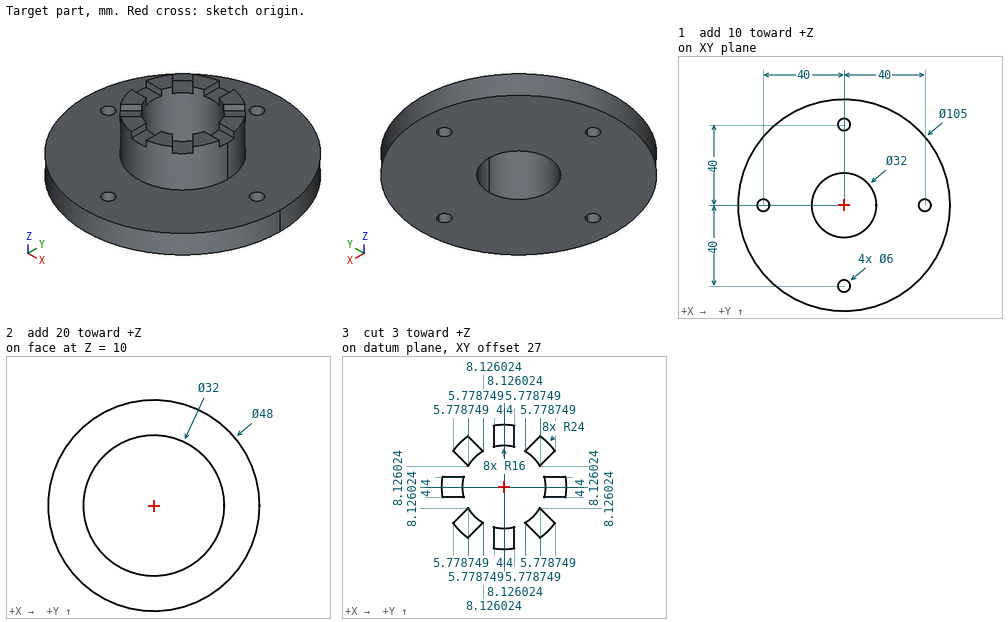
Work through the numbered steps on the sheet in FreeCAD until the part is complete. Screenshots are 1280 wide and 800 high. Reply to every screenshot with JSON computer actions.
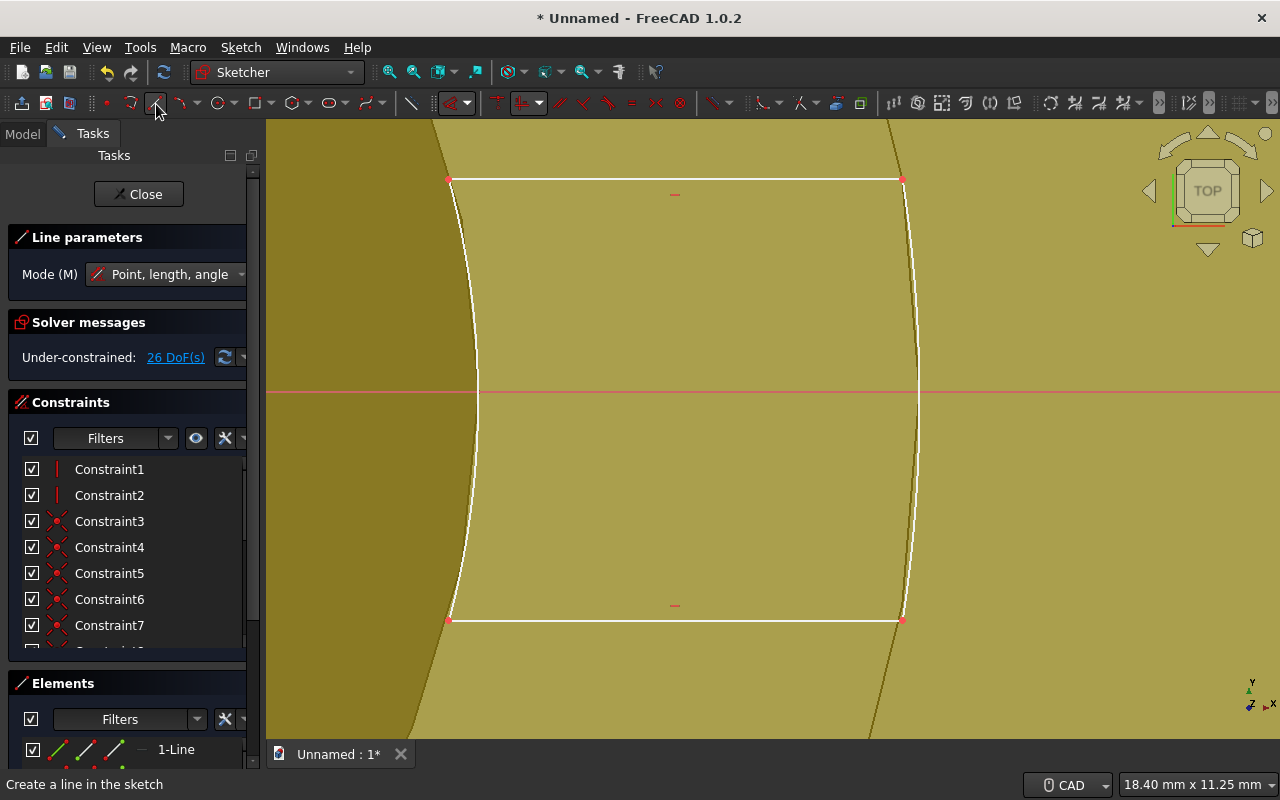
{"action": "scroll", "coordinate": [924, 436], "scroll_direction": "down", "scroll_amount": 9}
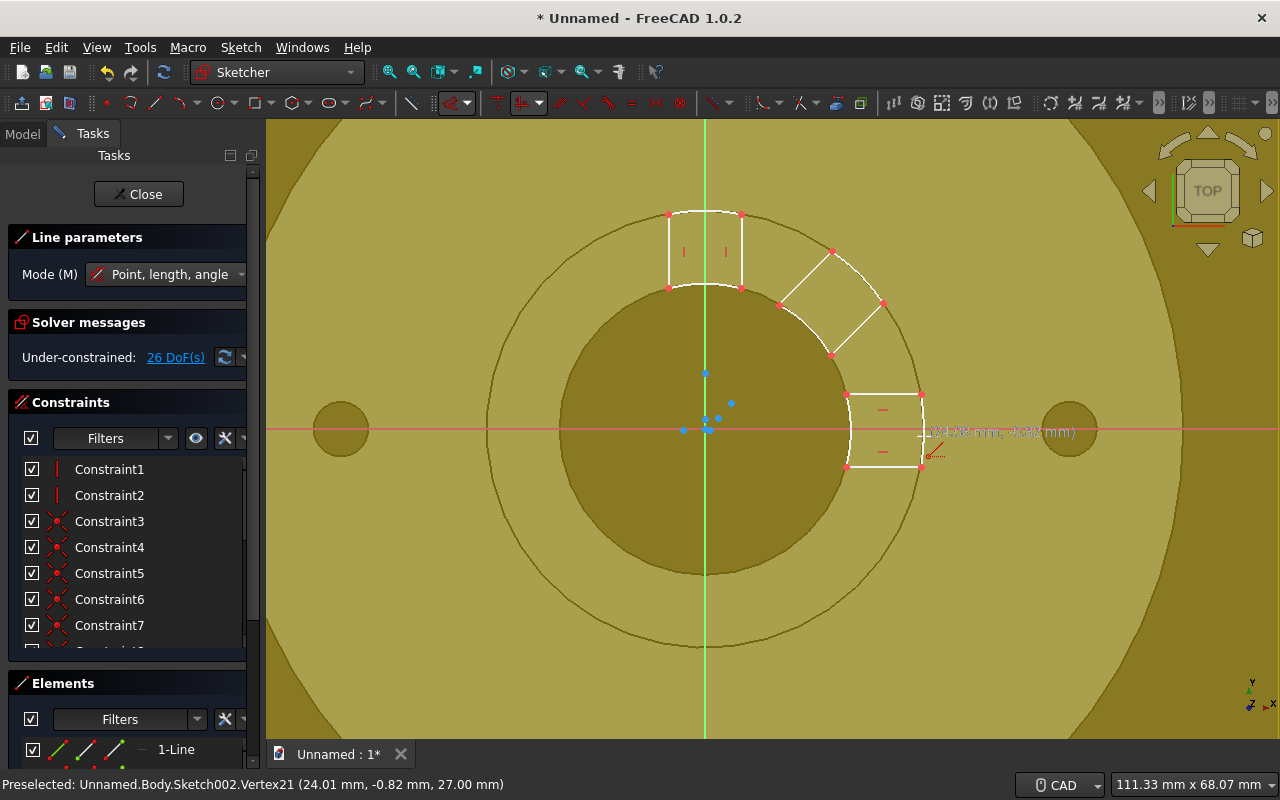
{"action": "left_click", "coordinate": [883, 556]}
{"action": "left_click", "coordinate": [831, 503]}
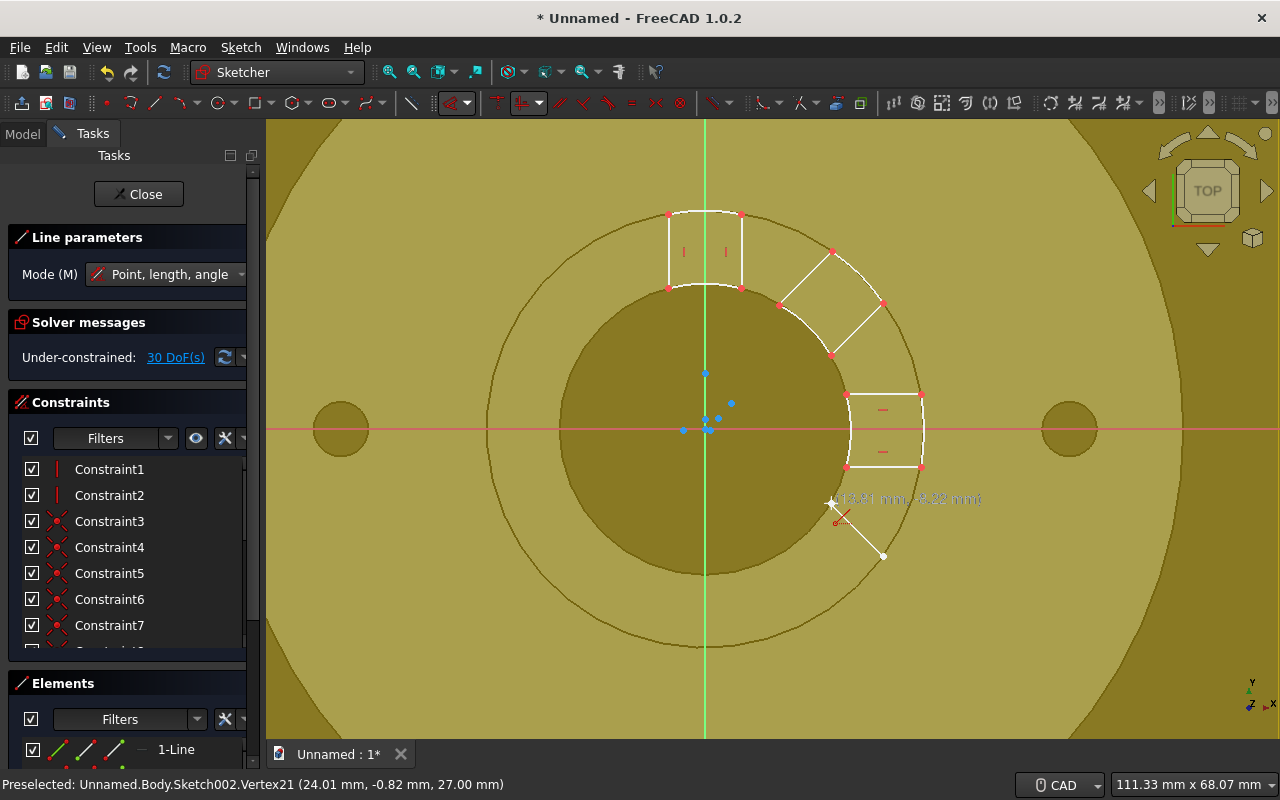
{"action": "left_click", "coordinate": [779, 555]}
{"action": "left_click", "coordinate": [832, 607]}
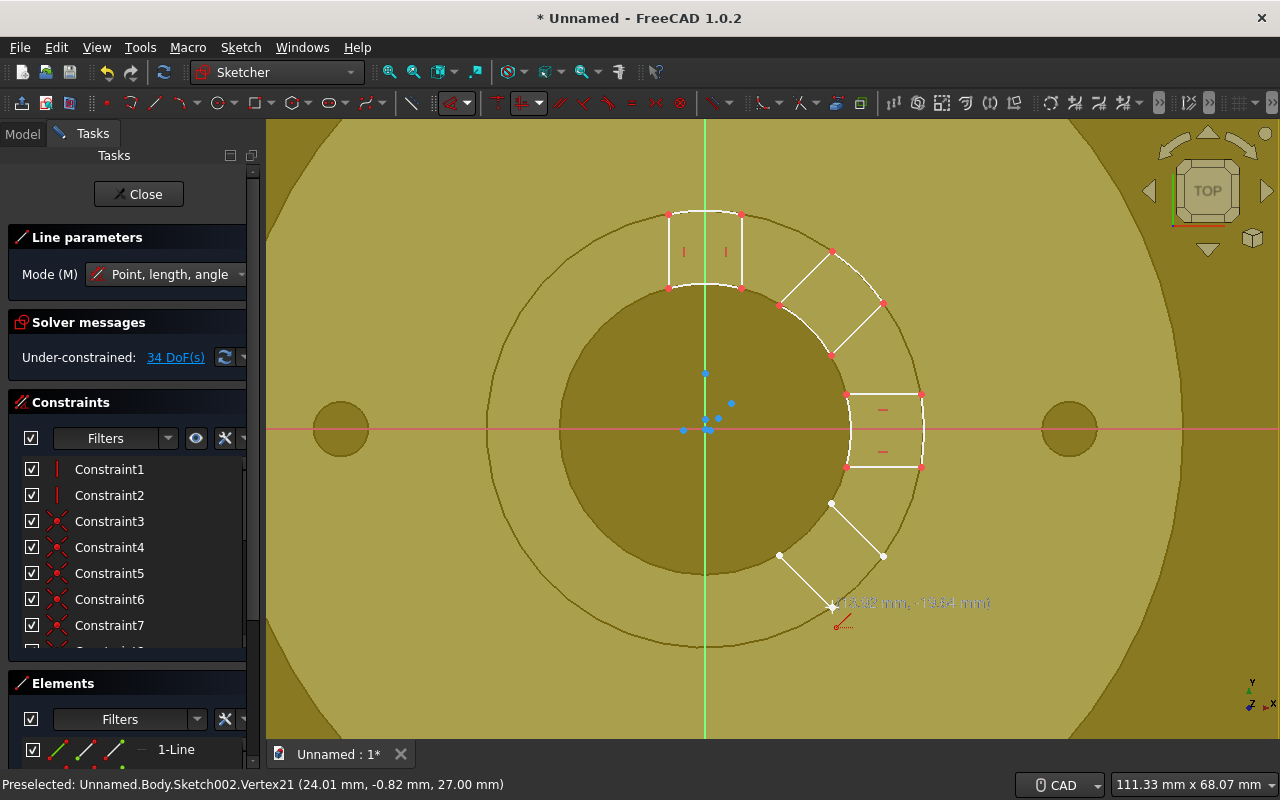
{"action": "left_click", "coordinate": [180, 104]}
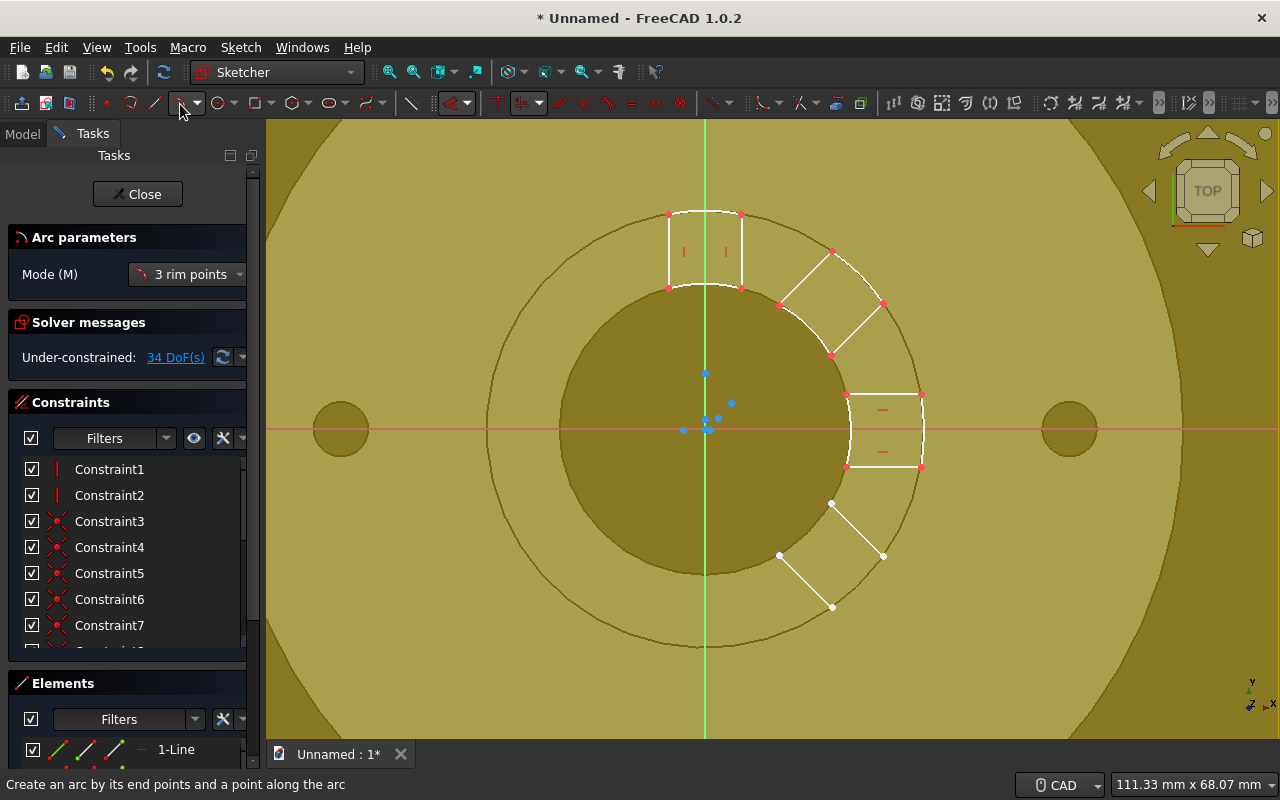
{"action": "left_click", "coordinate": [831, 504]}
{"action": "left_click", "coordinate": [779, 556]}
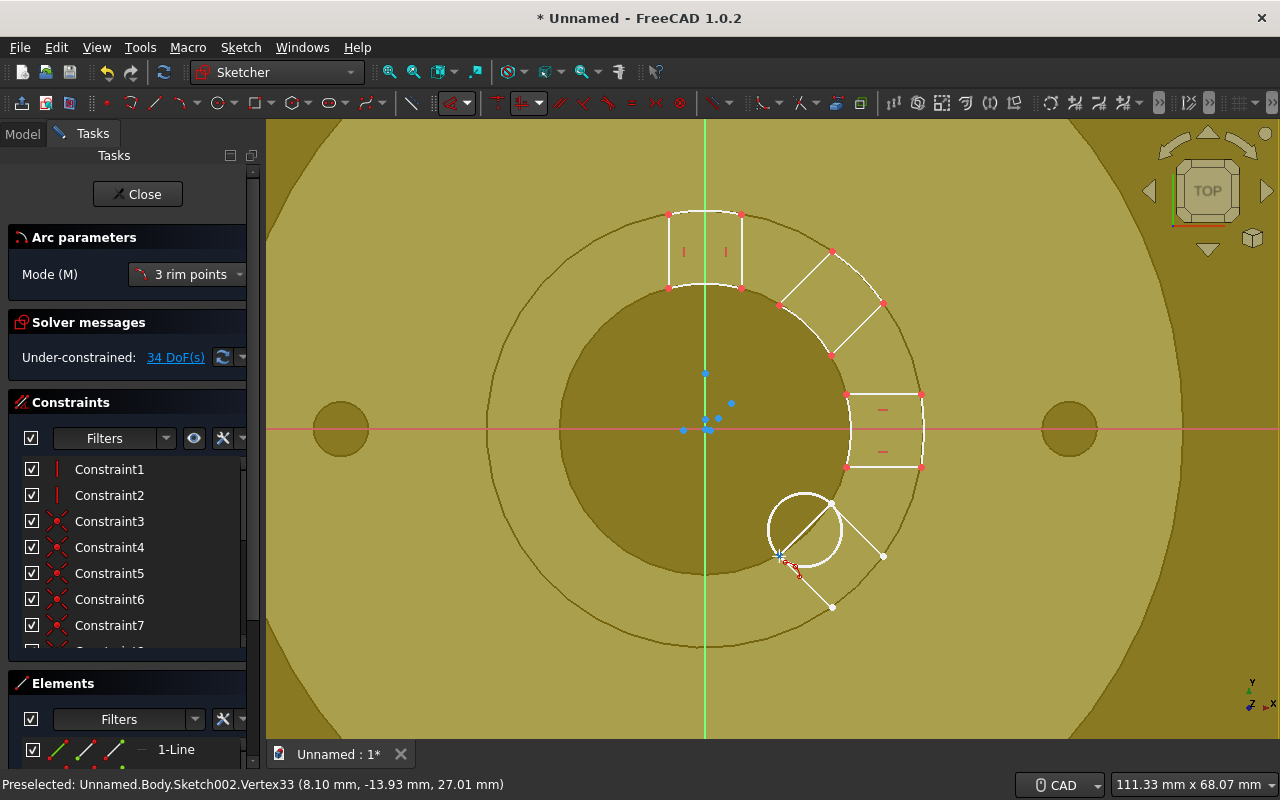
{"action": "scroll", "coordinate": [808, 532], "scroll_direction": "up", "scroll_amount": 7}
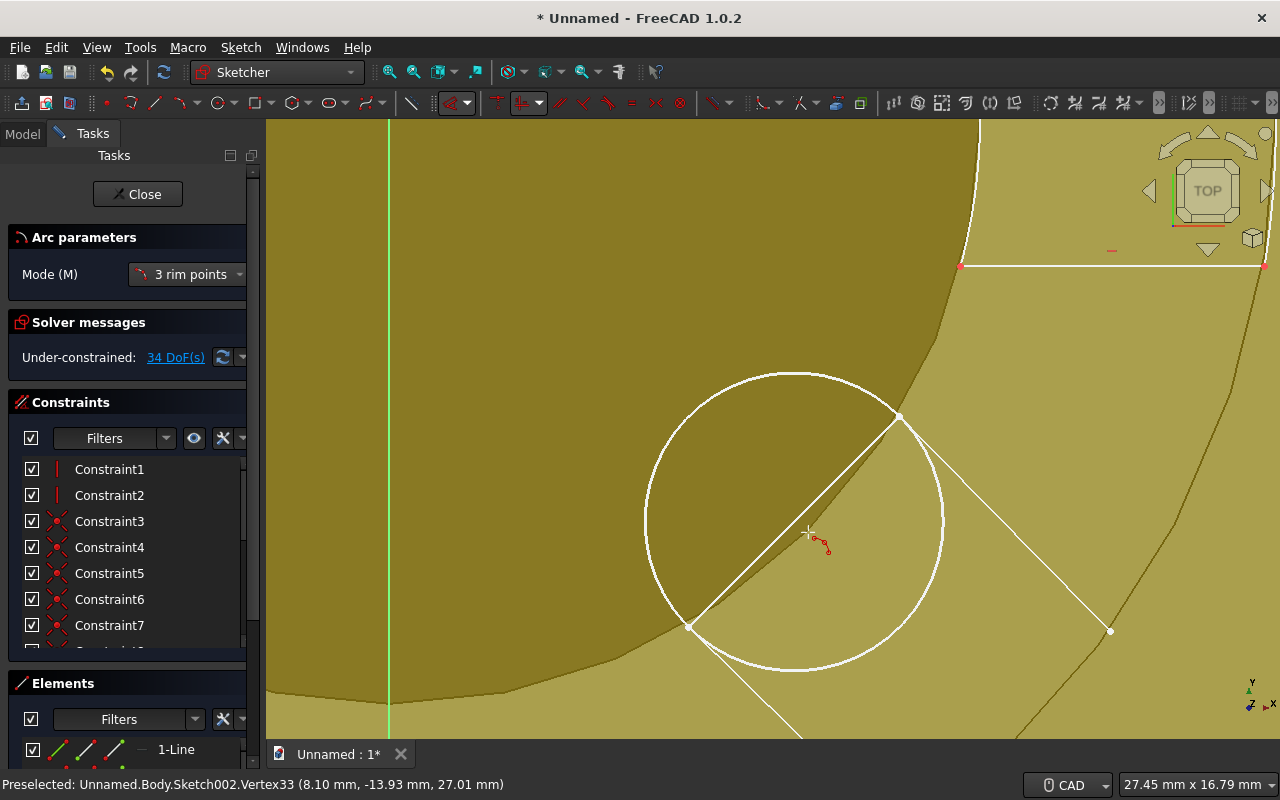
{"action": "left_click", "coordinate": [807, 531]}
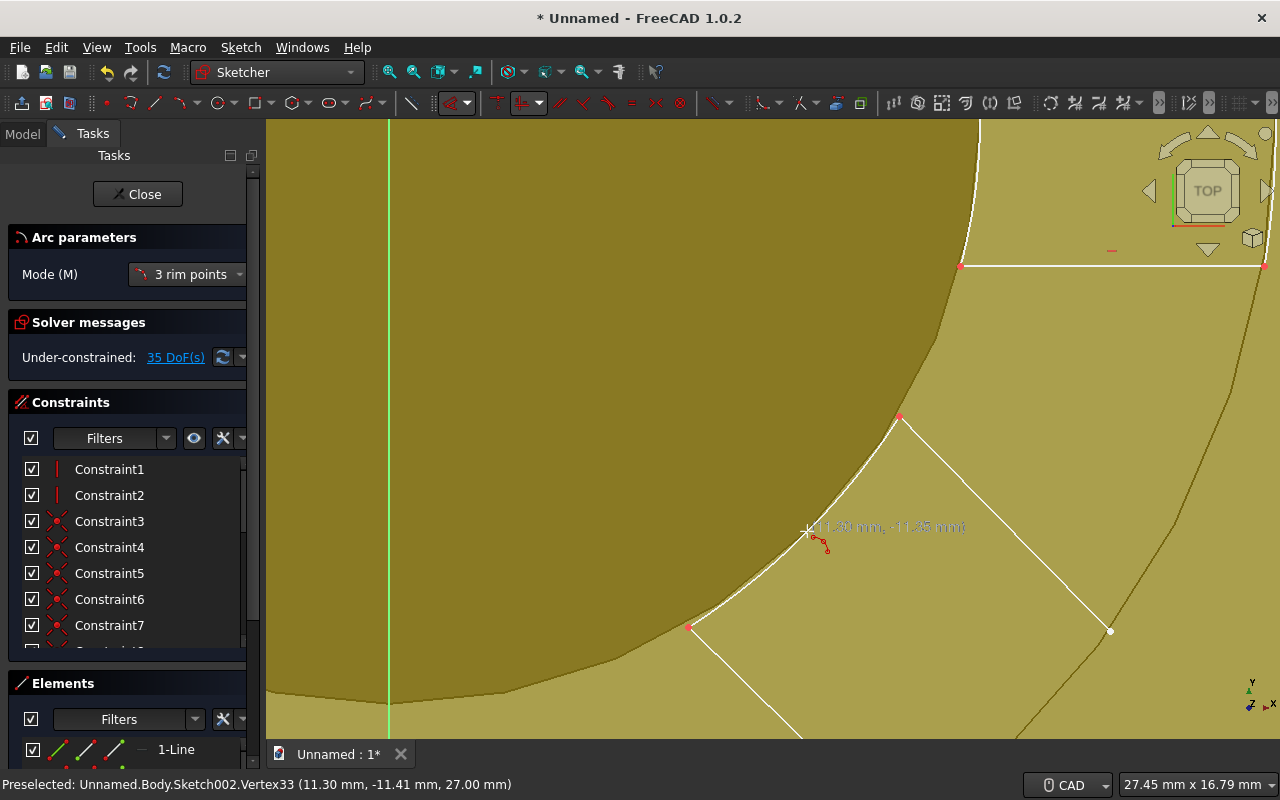
{"action": "scroll", "coordinate": [808, 532], "scroll_direction": "down", "scroll_amount": 7}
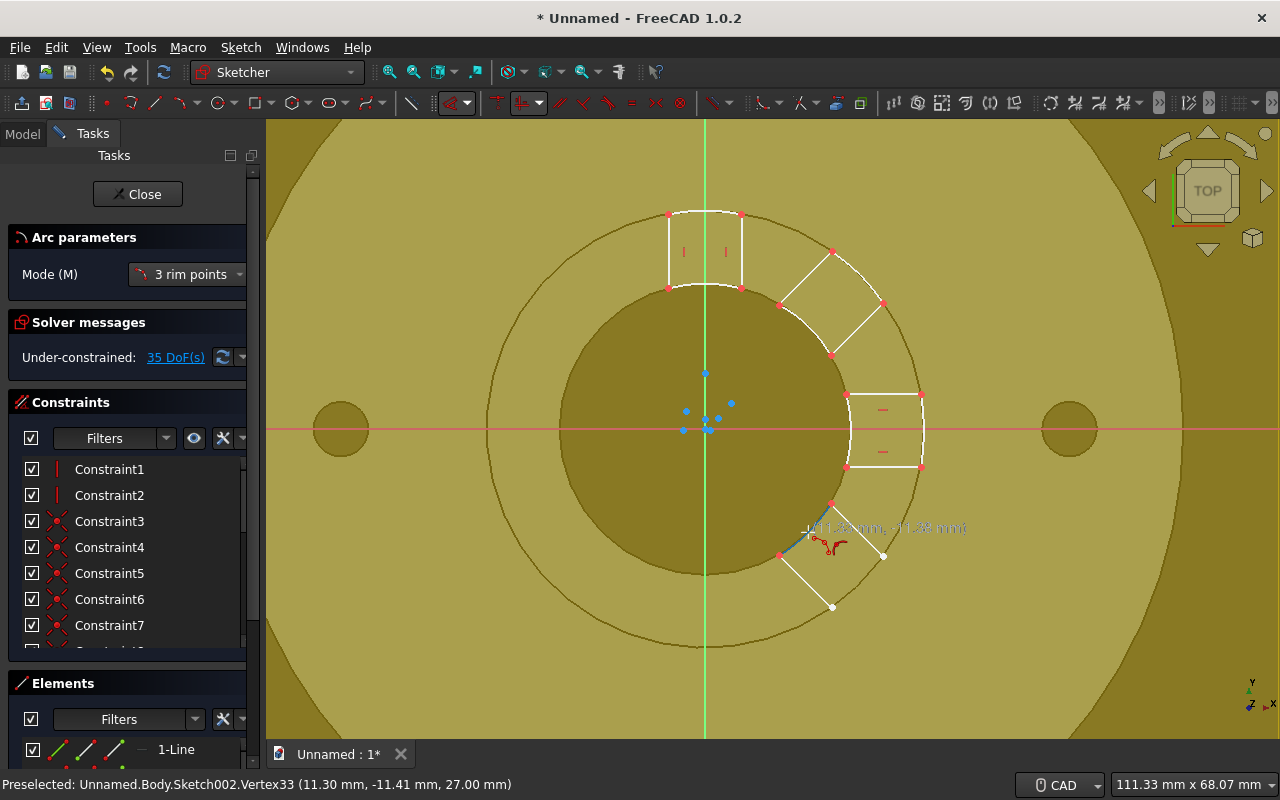
{"action": "left_click", "coordinate": [832, 608]}
{"action": "left_click", "coordinate": [883, 557]}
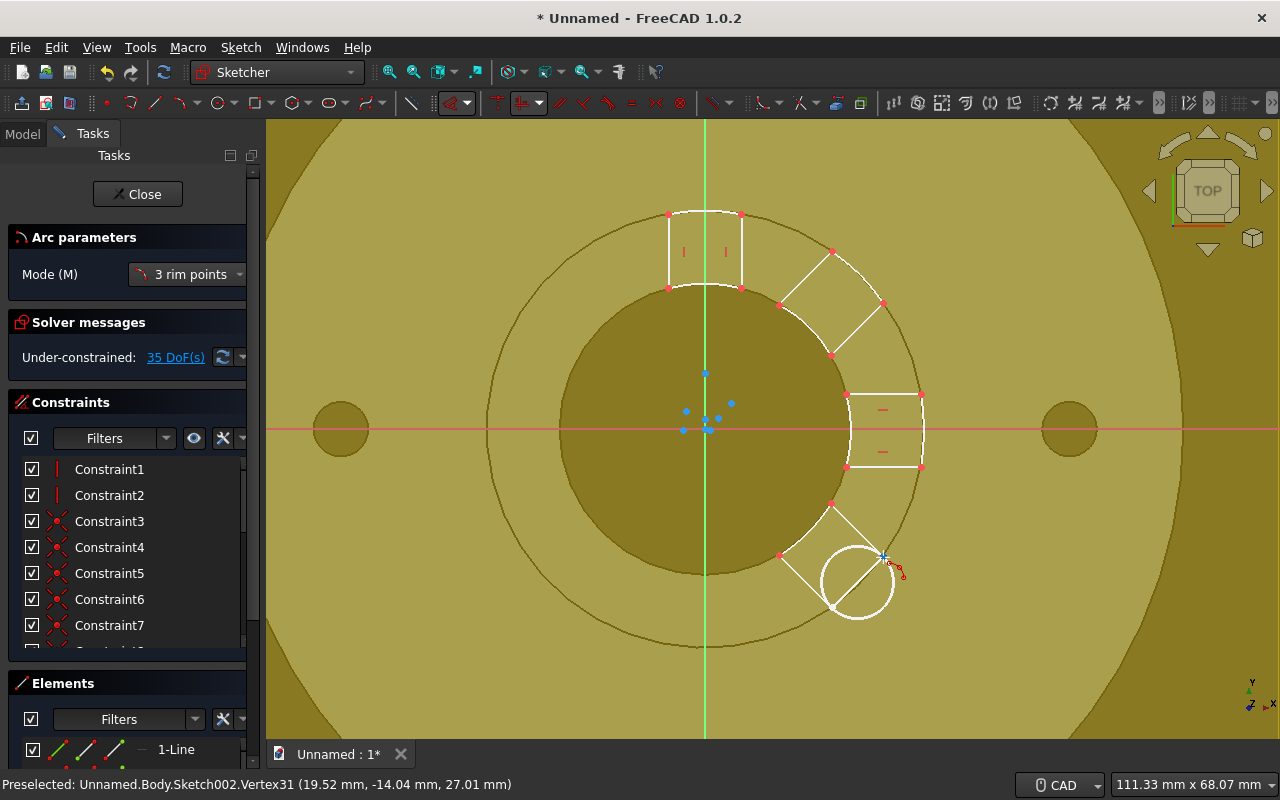
{"action": "scroll", "coordinate": [860, 584], "scroll_direction": "up", "scroll_amount": 9}